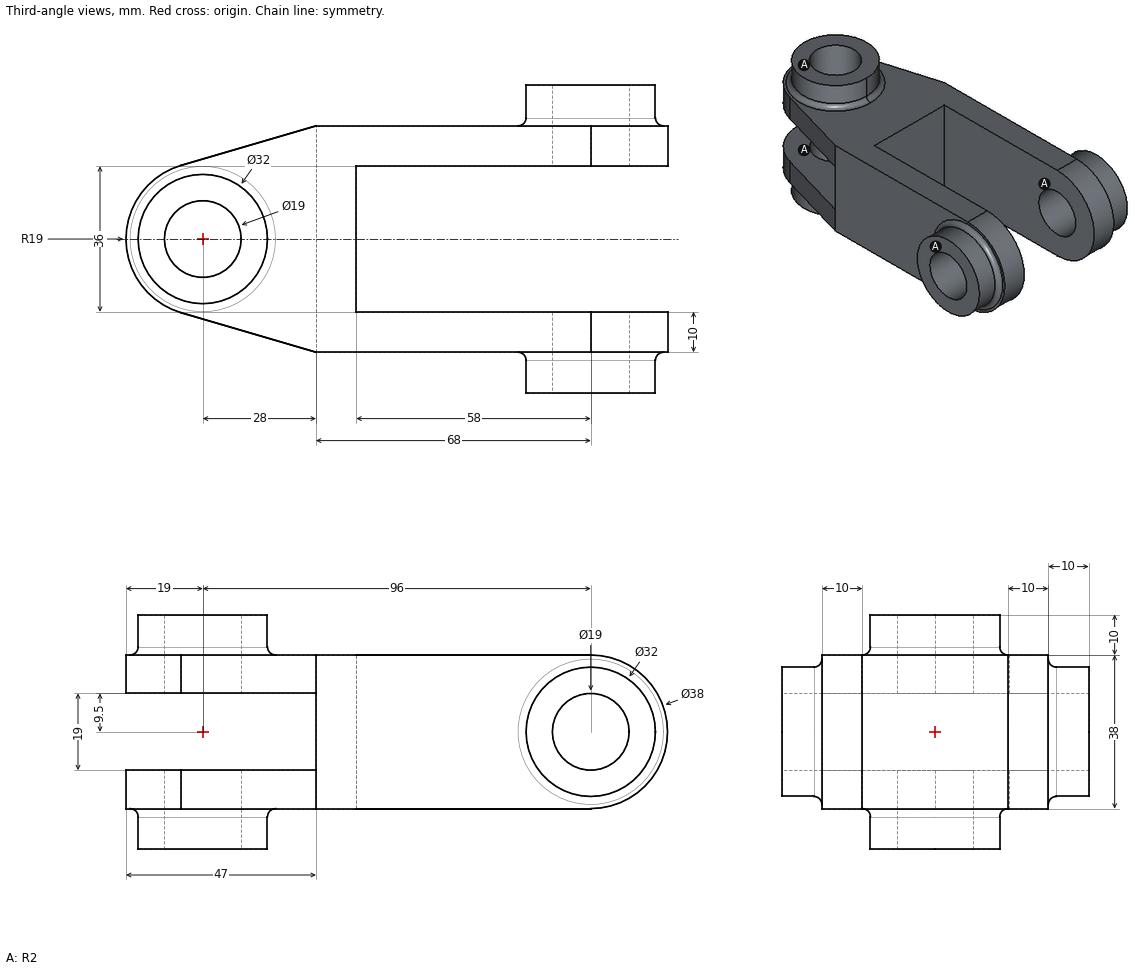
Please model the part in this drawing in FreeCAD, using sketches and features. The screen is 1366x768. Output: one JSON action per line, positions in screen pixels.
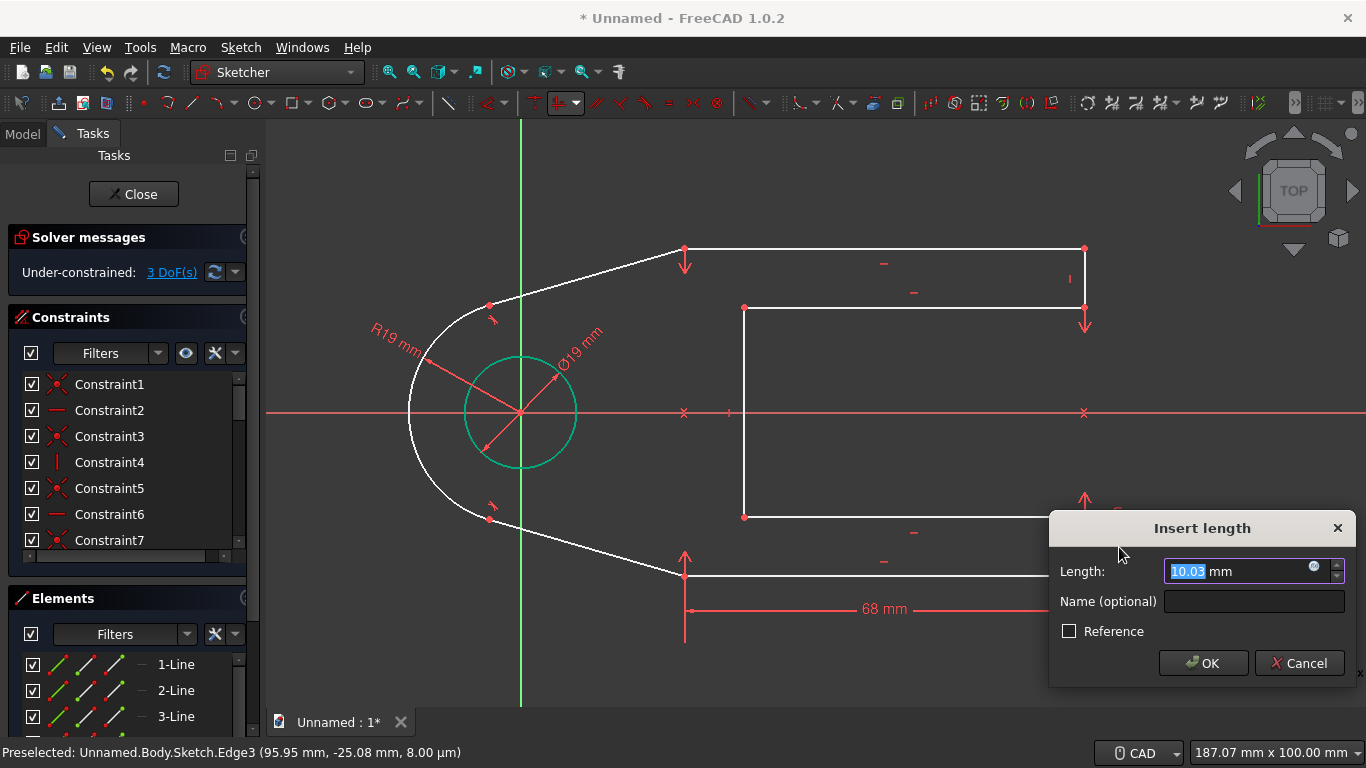
{"action": "type", "text": "10"}
{"action": "key", "text": "Return"}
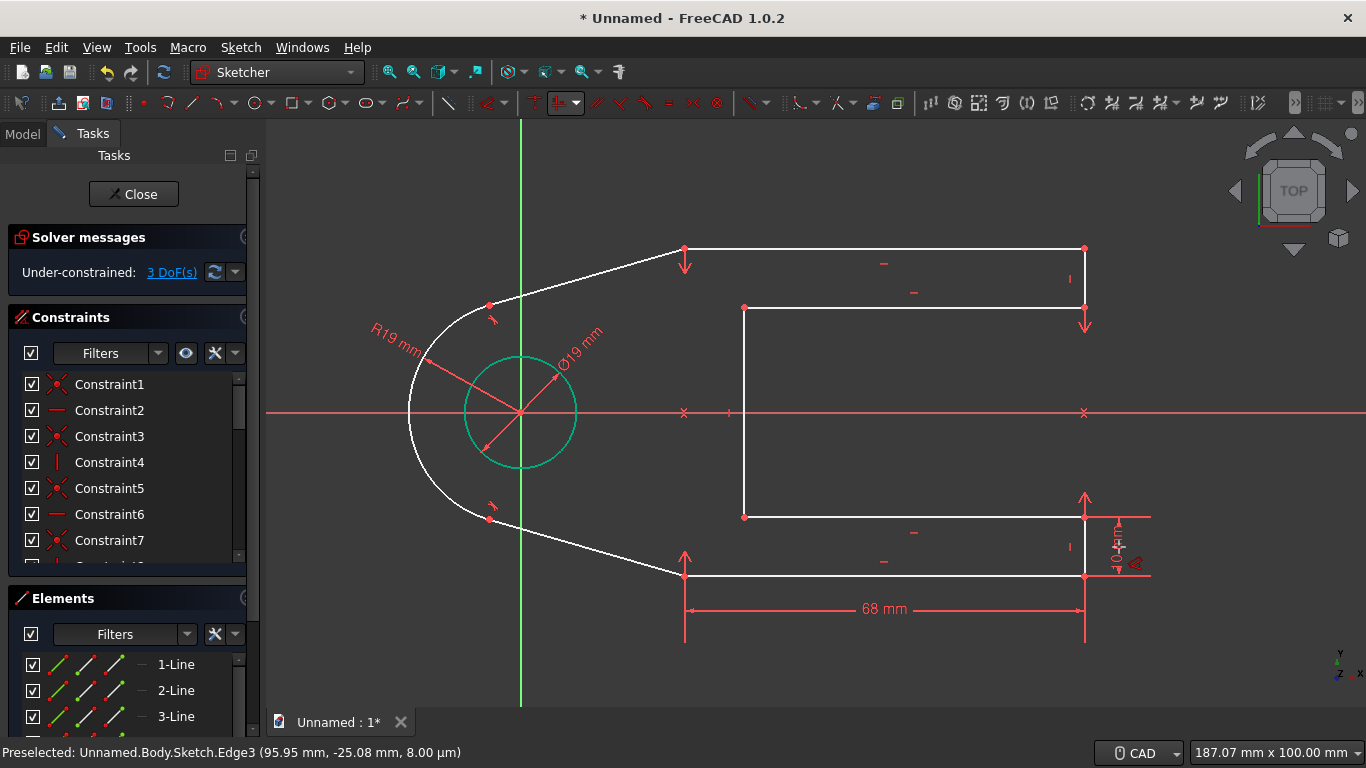
{"action": "left_click", "coordinate": [983, 517]}
{"action": "left_click", "coordinate": [914, 551]}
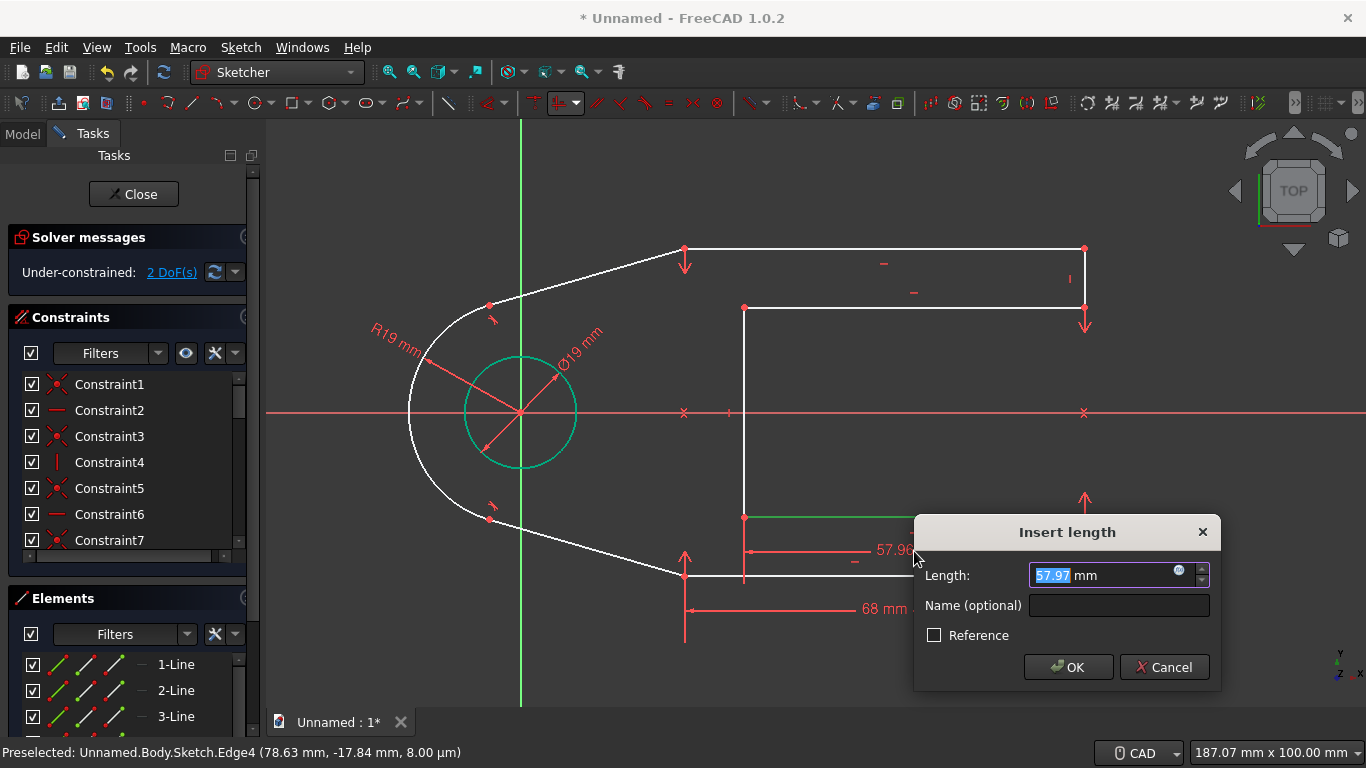
{"action": "type", "text": "58"}
{"action": "key", "text": "Return"}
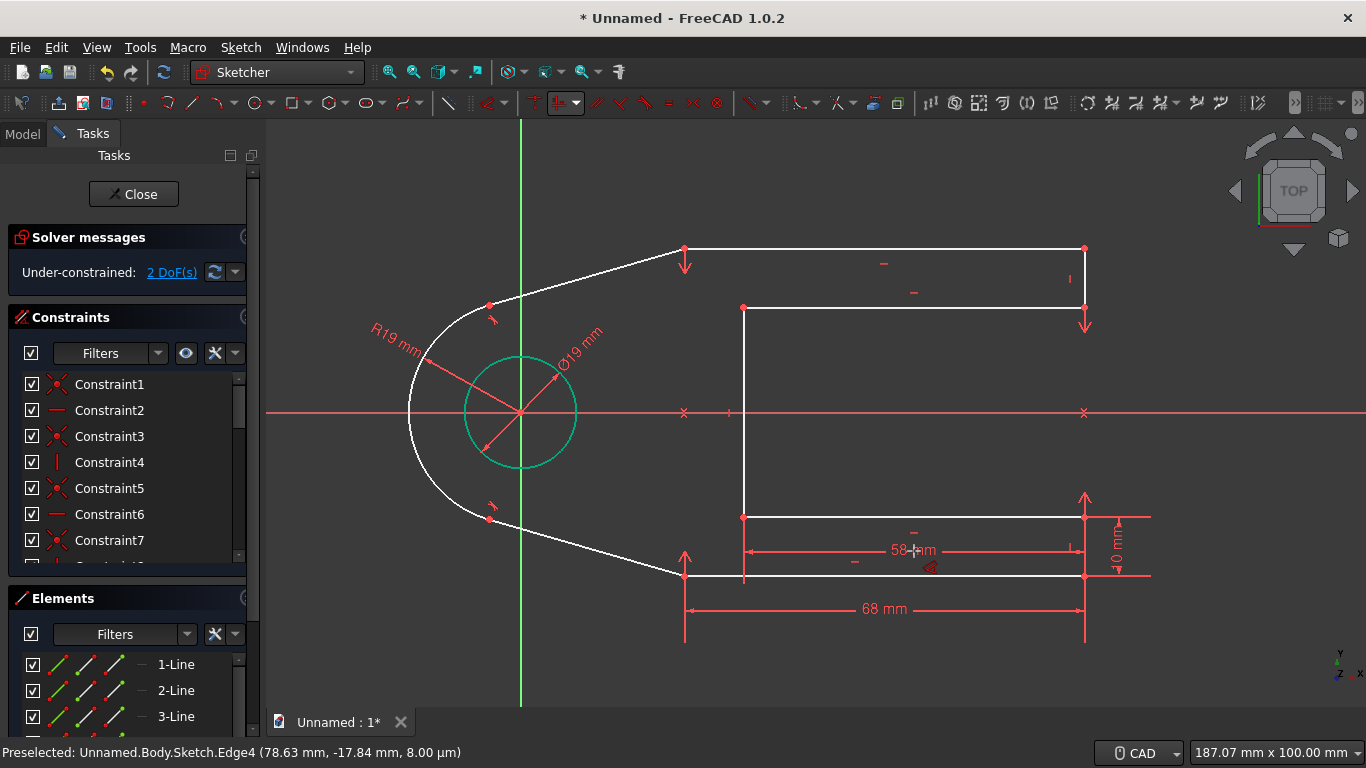
{"action": "left_click", "coordinate": [744, 454]}
{"action": "left_click", "coordinate": [710, 364]}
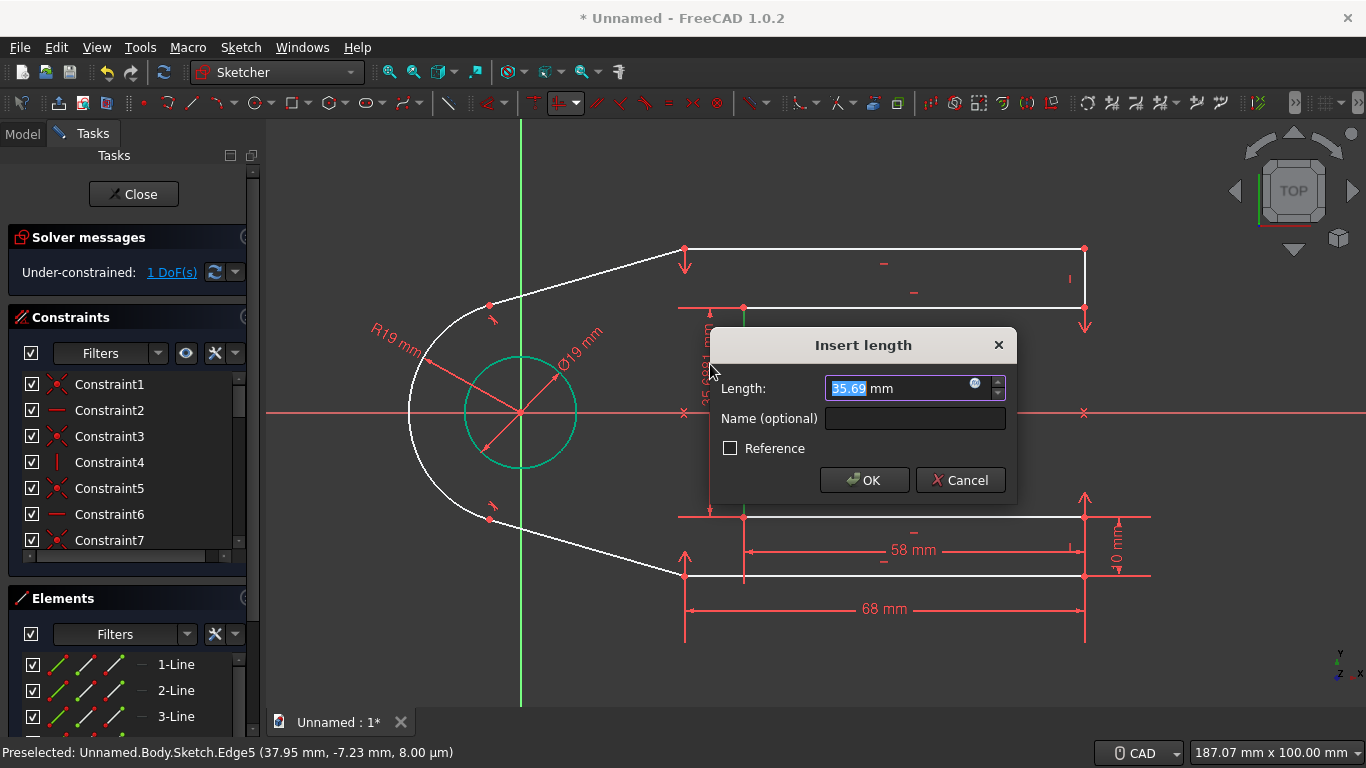
{"action": "type", "text": "36"}
{"action": "key", "text": "Return"}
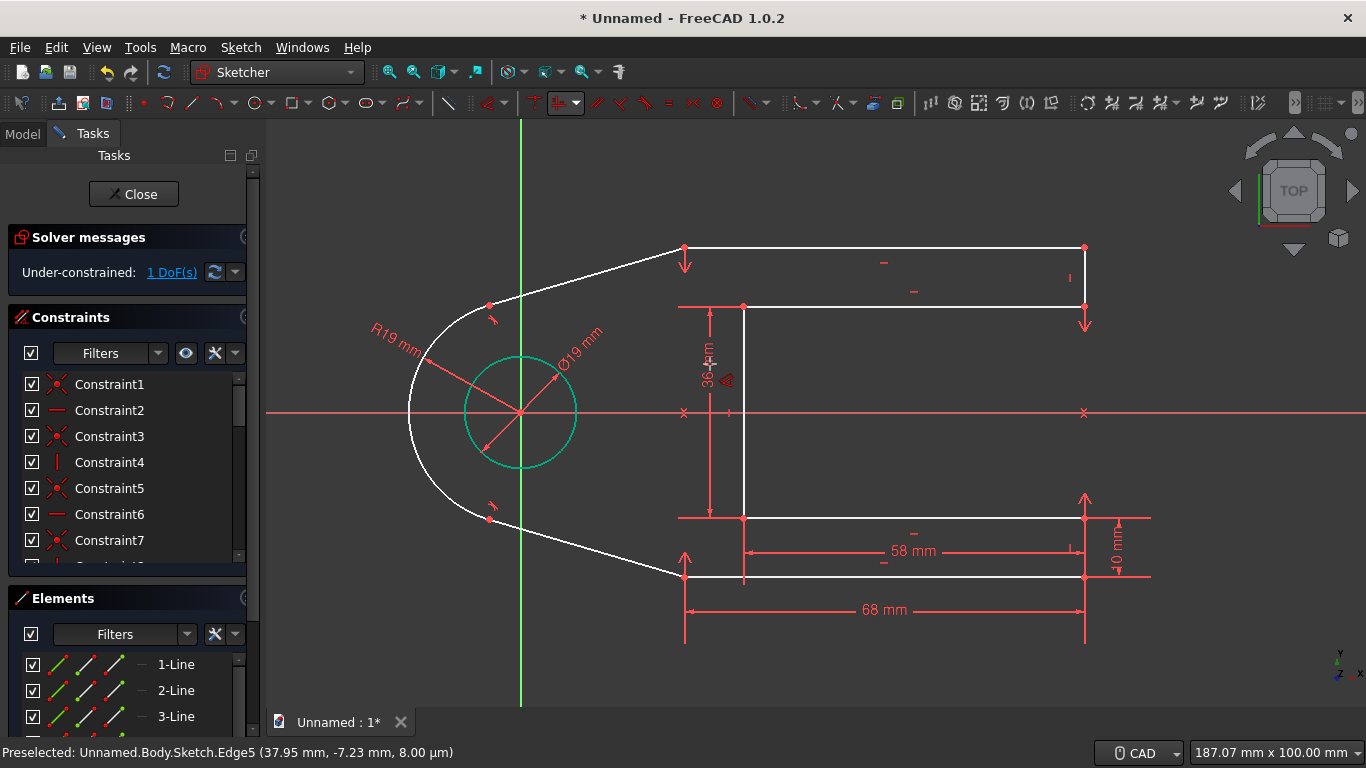
{"action": "left_click", "coordinate": [685, 577]}
{"action": "left_click", "coordinate": [603, 611]}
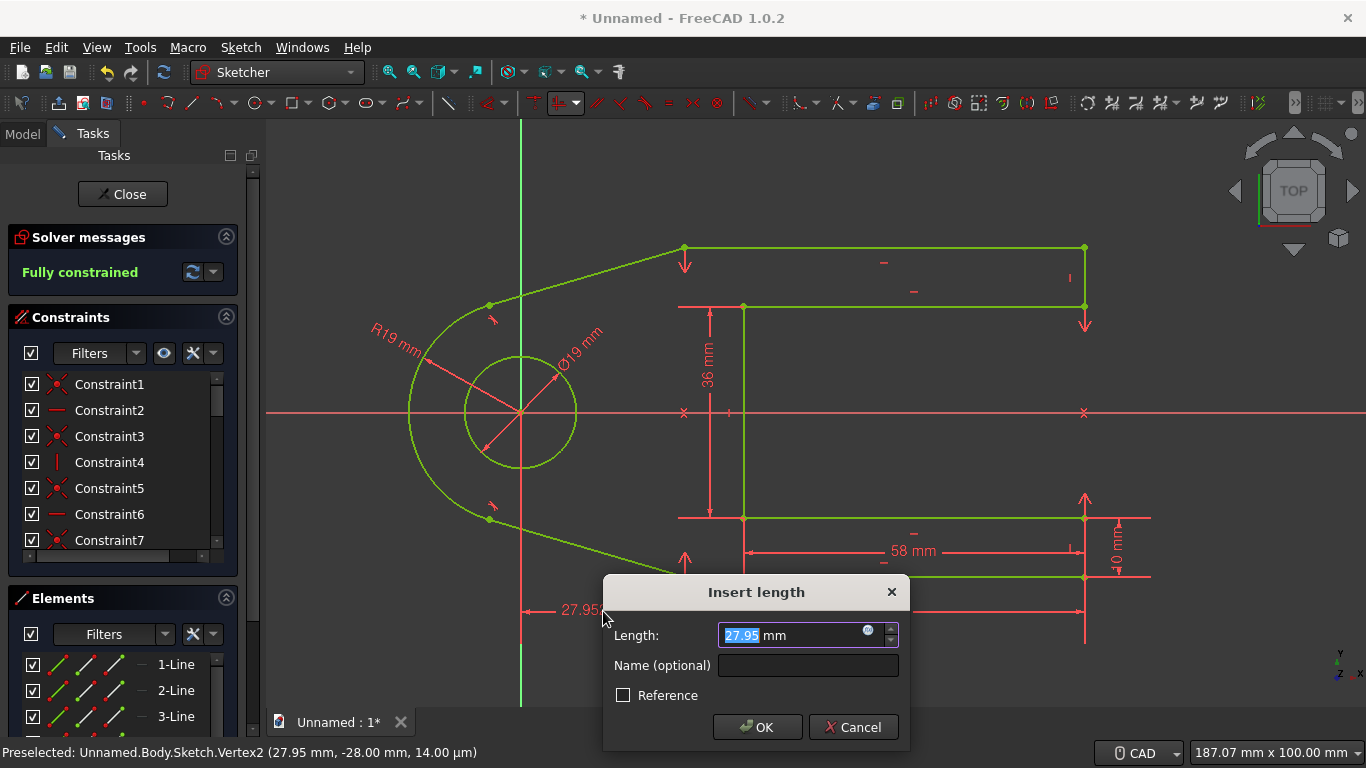
{"action": "type", "text": "28"}
{"action": "key", "text": "Return"}
{"action": "key", "text": "Escape"}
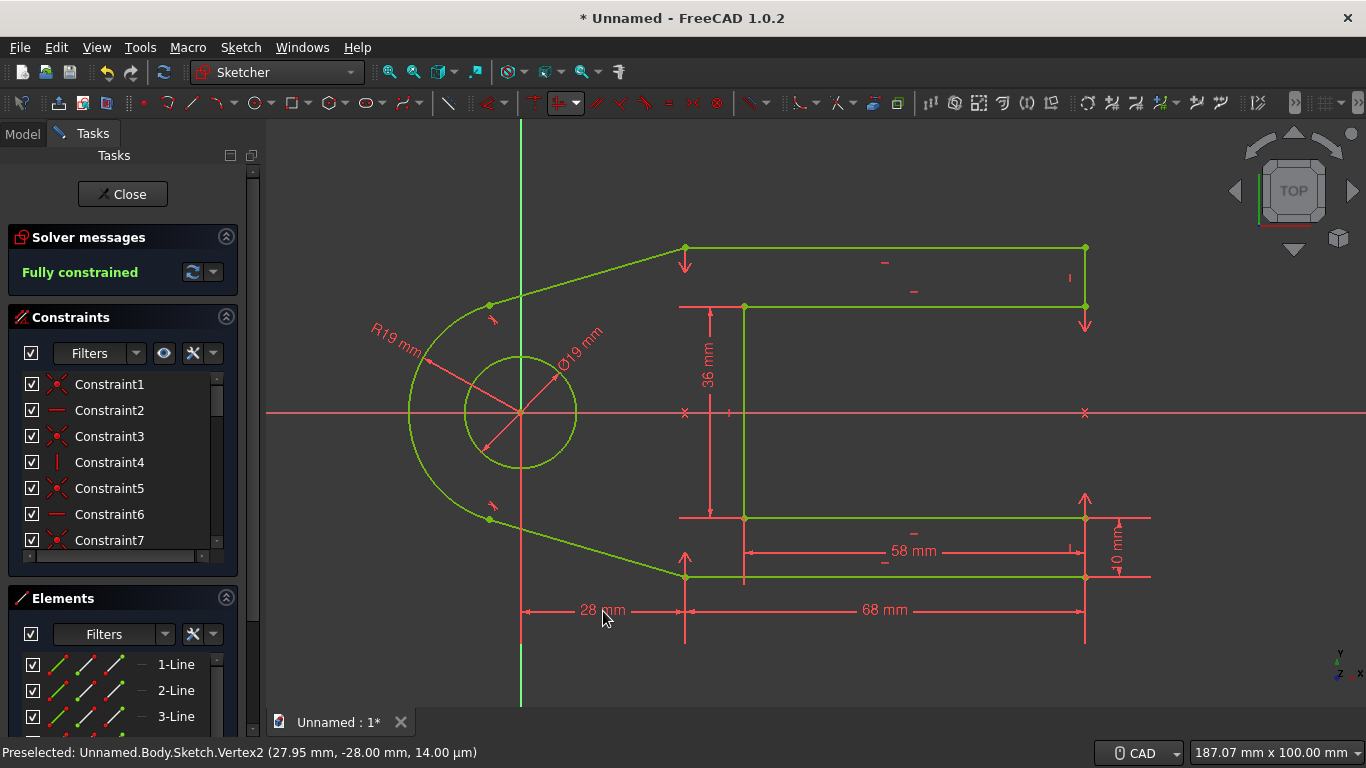
{"action": "left_click", "coordinate": [123, 194]}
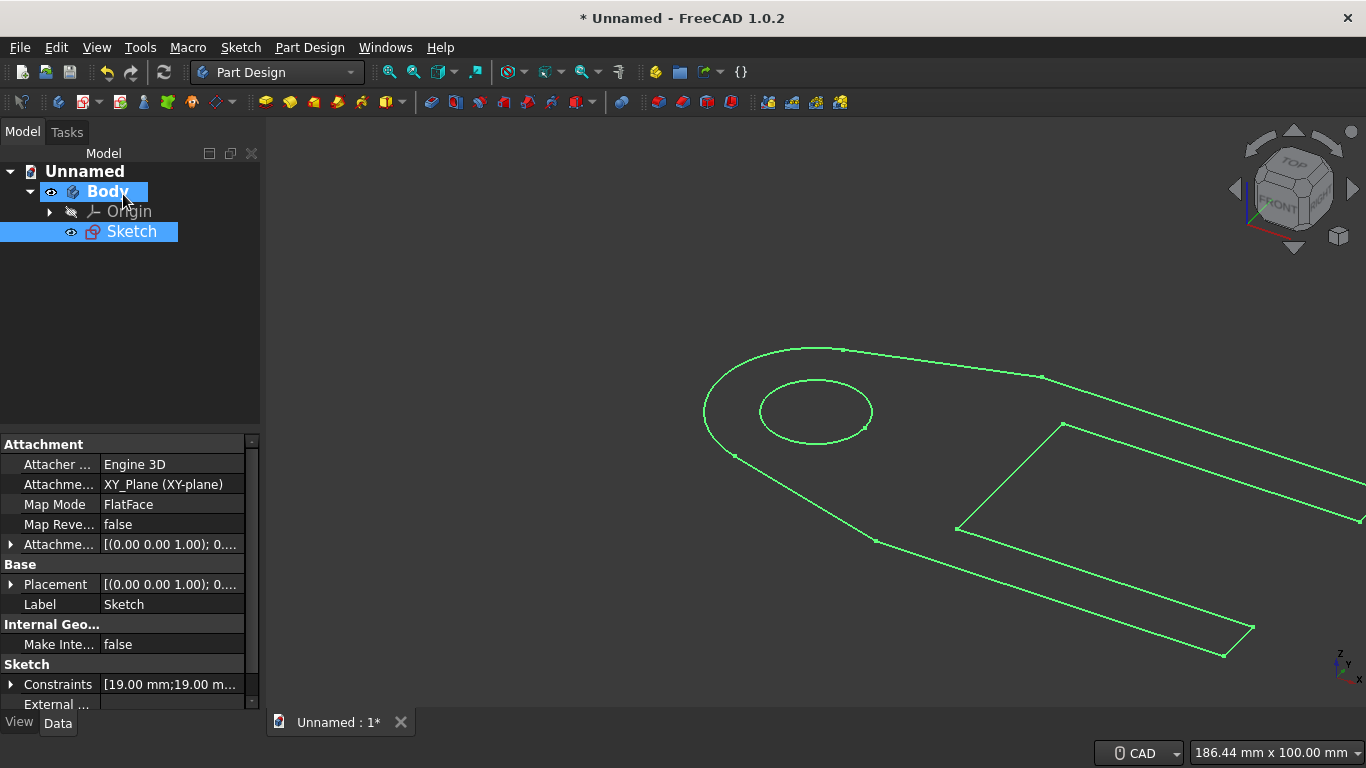
{"action": "left_click", "coordinate": [266, 102]}